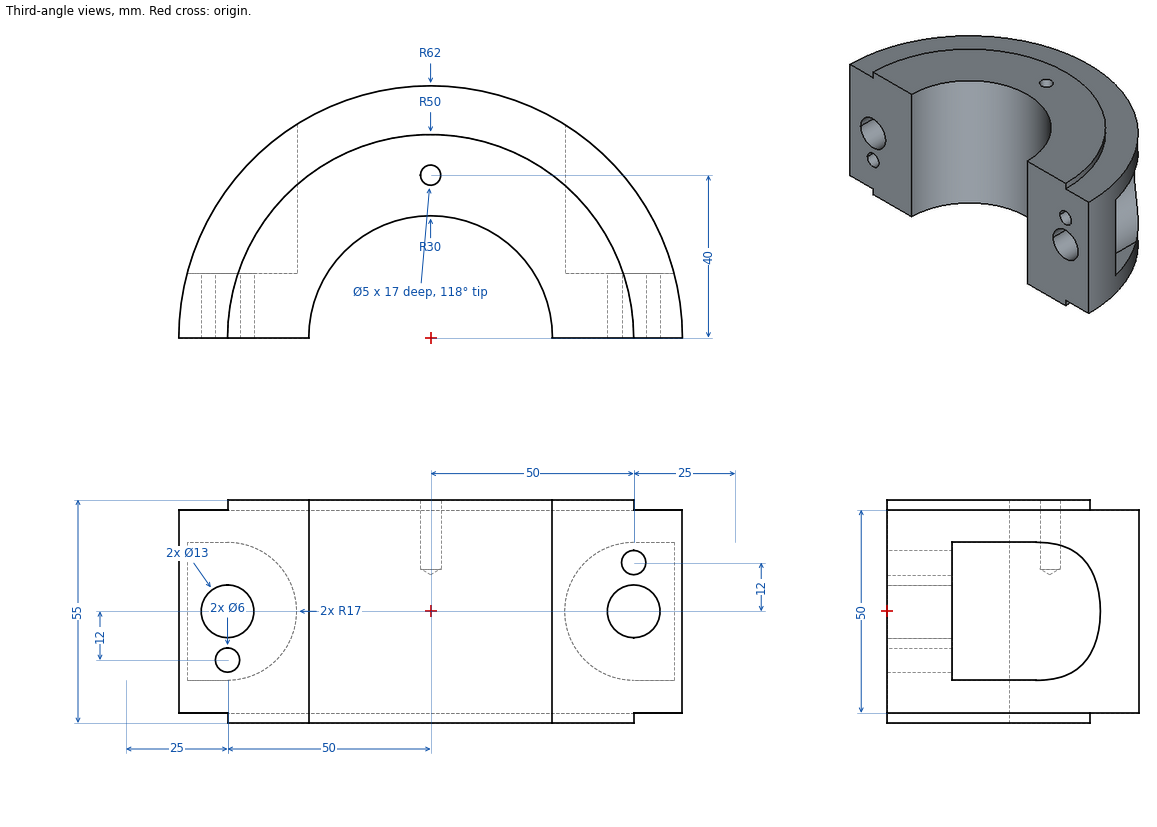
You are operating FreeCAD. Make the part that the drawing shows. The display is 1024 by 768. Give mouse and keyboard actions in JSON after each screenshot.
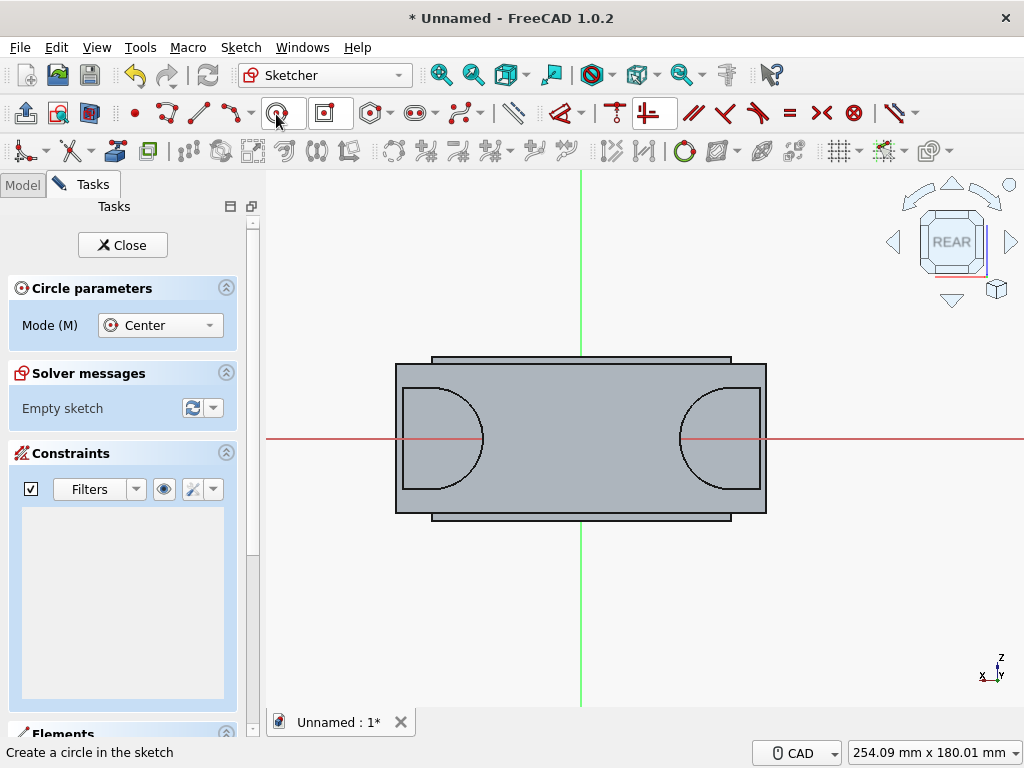
{"action": "left_click", "coordinate": [731, 439]}
{"action": "mouse_move", "coordinate": [737, 420]}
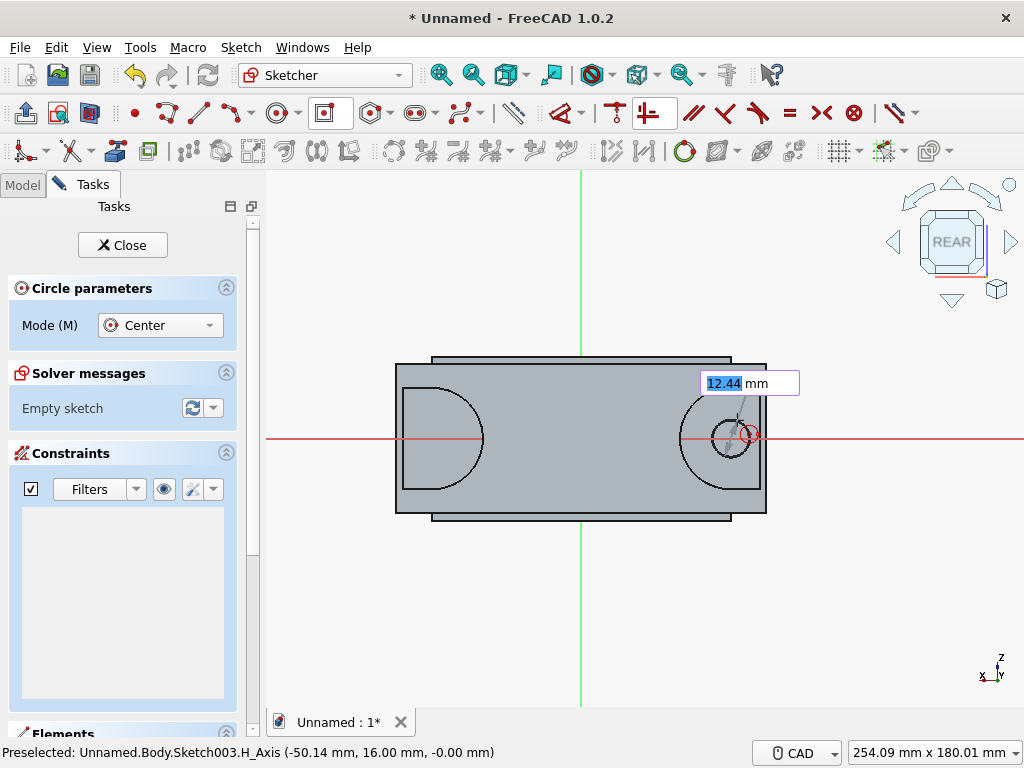
{"action": "type", "text": "13"}
{"action": "key", "text": "Return"}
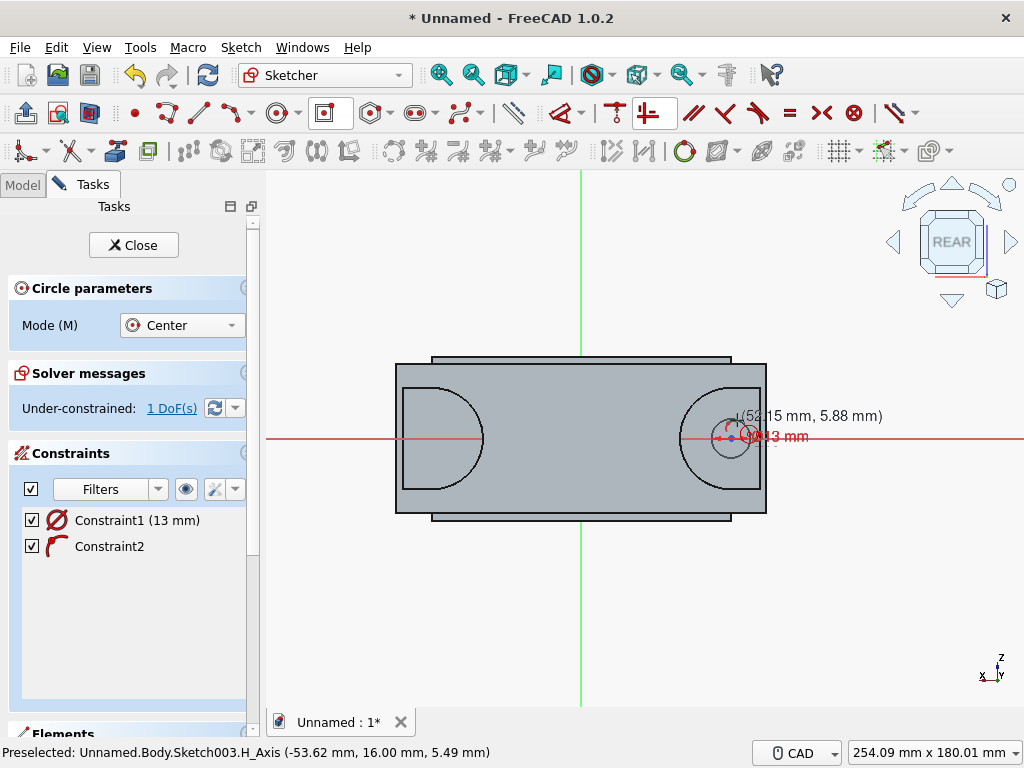
{"action": "scroll", "coordinate": [731, 474], "scroll_direction": "up", "scroll_amount": 5}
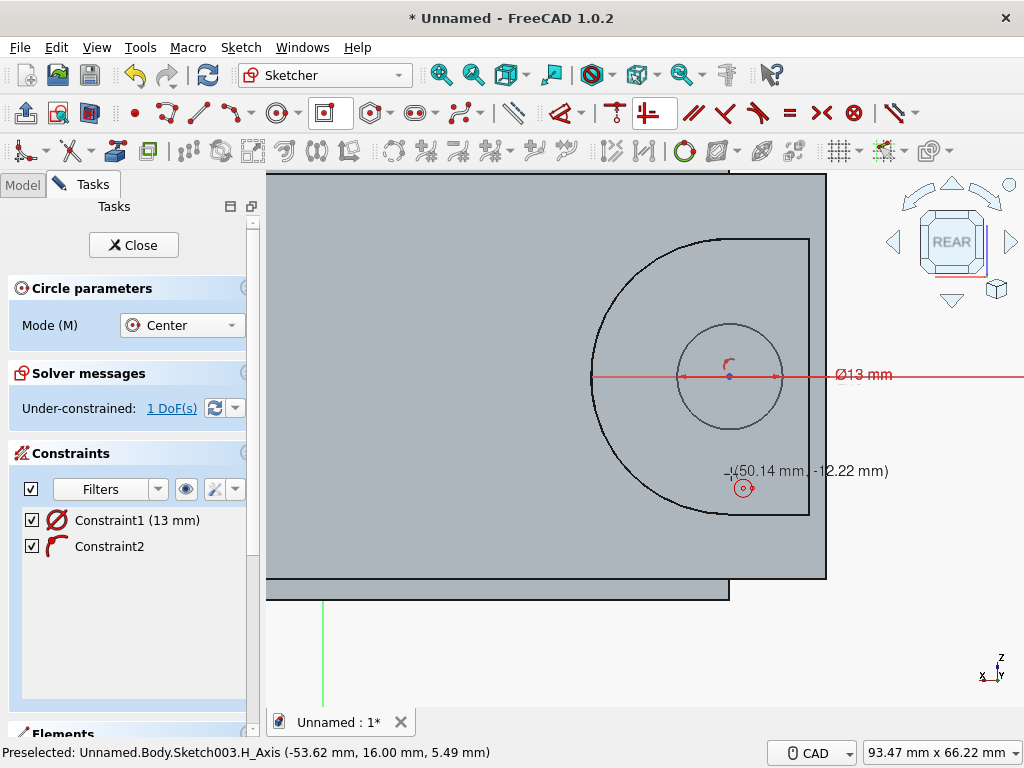
{"action": "left_click", "coordinate": [729, 474]}
{"action": "mouse_move", "coordinate": [746, 457]}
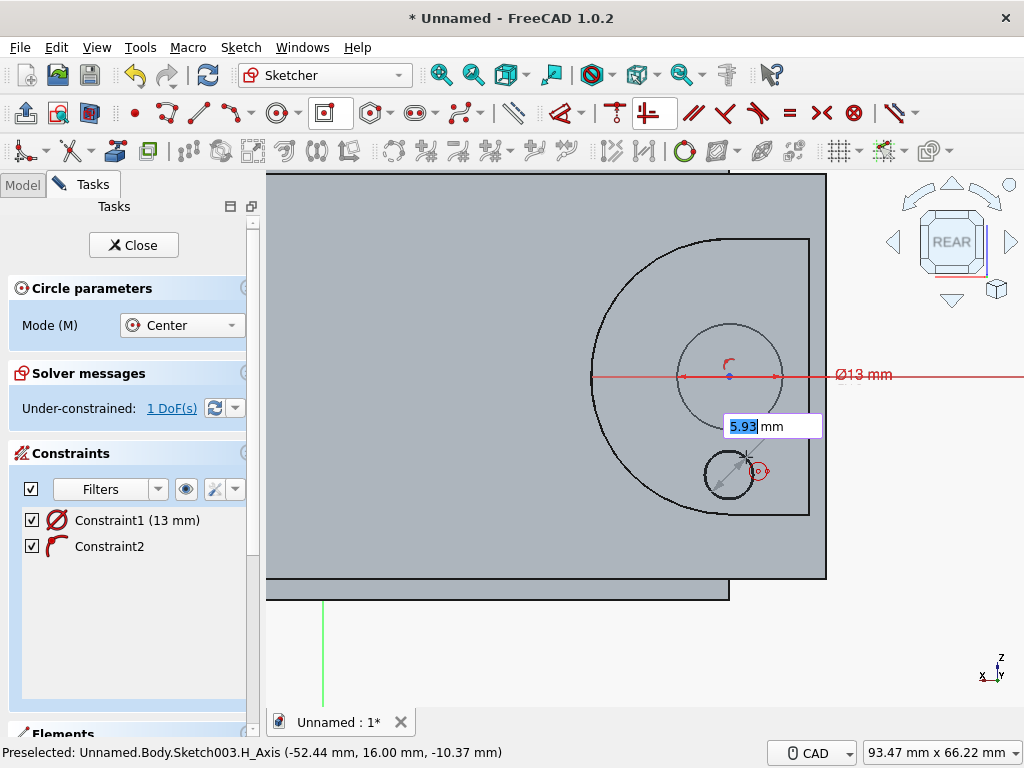
{"action": "type", "text": "6"}
{"action": "key", "text": "Return"}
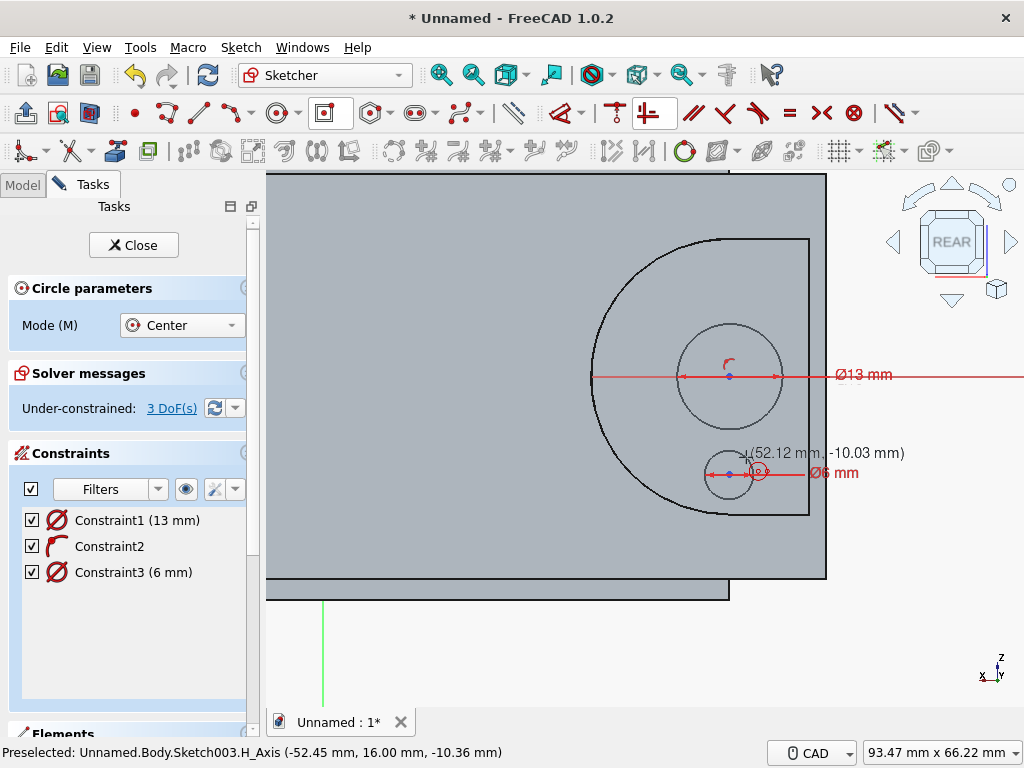
{"action": "scroll", "coordinate": [783, 489], "scroll_direction": "down", "scroll_amount": 4}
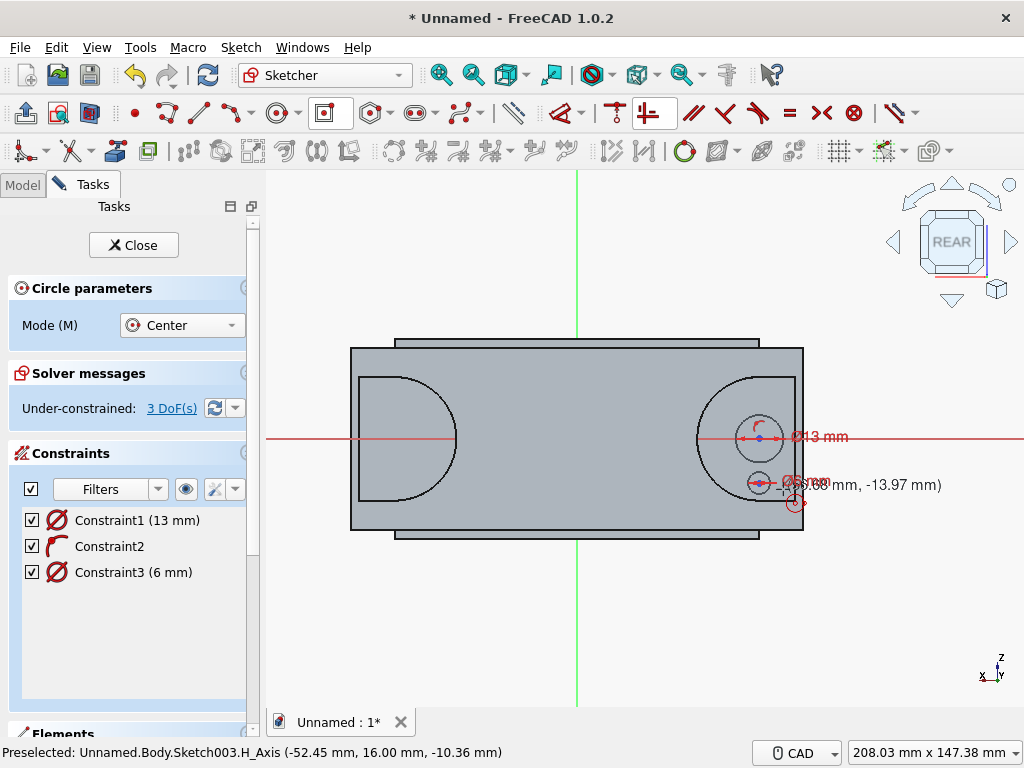
{"action": "left_click", "coordinate": [395, 439]}
{"action": "mouse_move", "coordinate": [411, 422]}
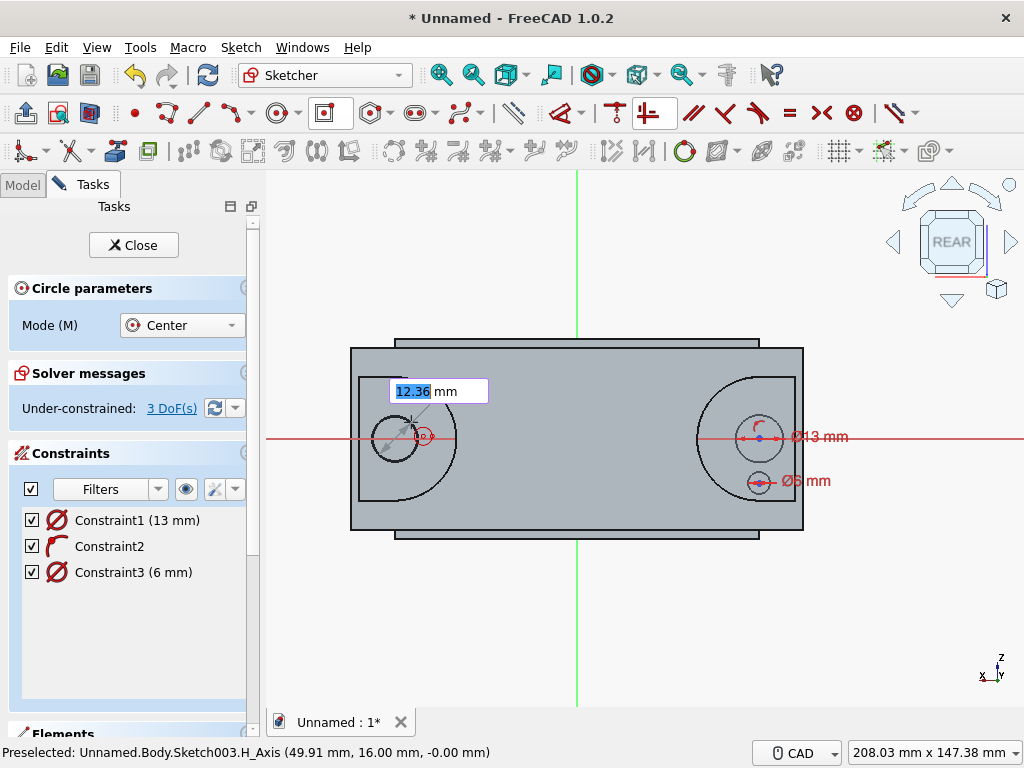
{"action": "type", "text": "13"}
{"action": "key", "text": "Return"}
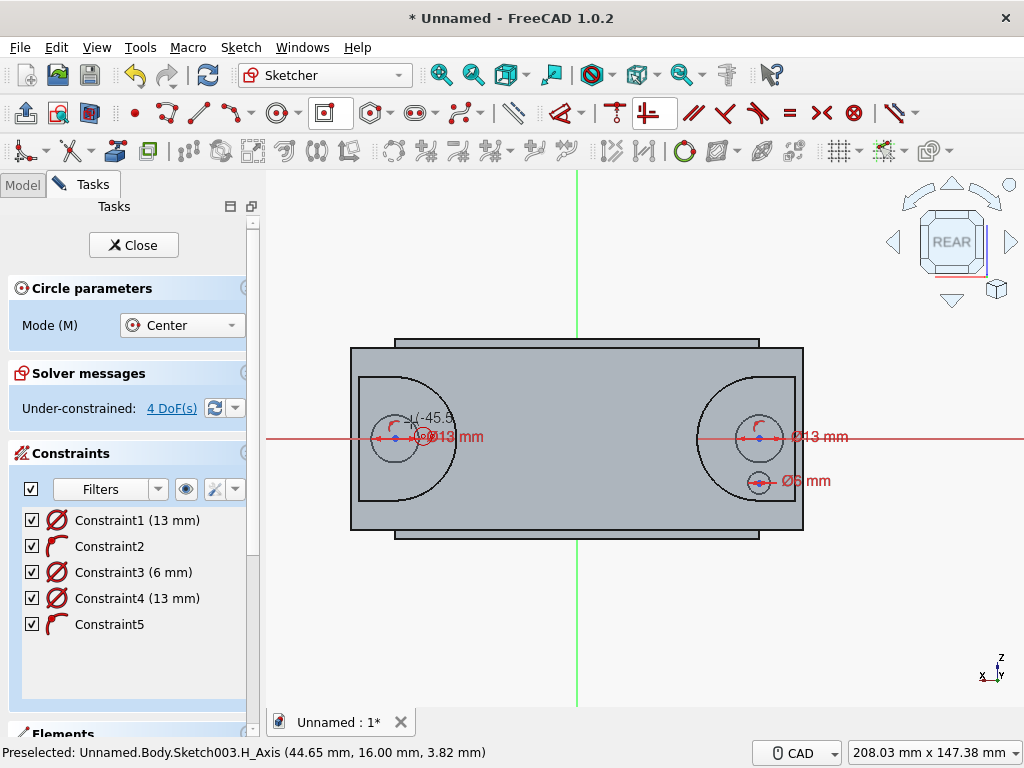
{"action": "scroll", "coordinate": [395, 395], "scroll_direction": "up", "scroll_amount": 4}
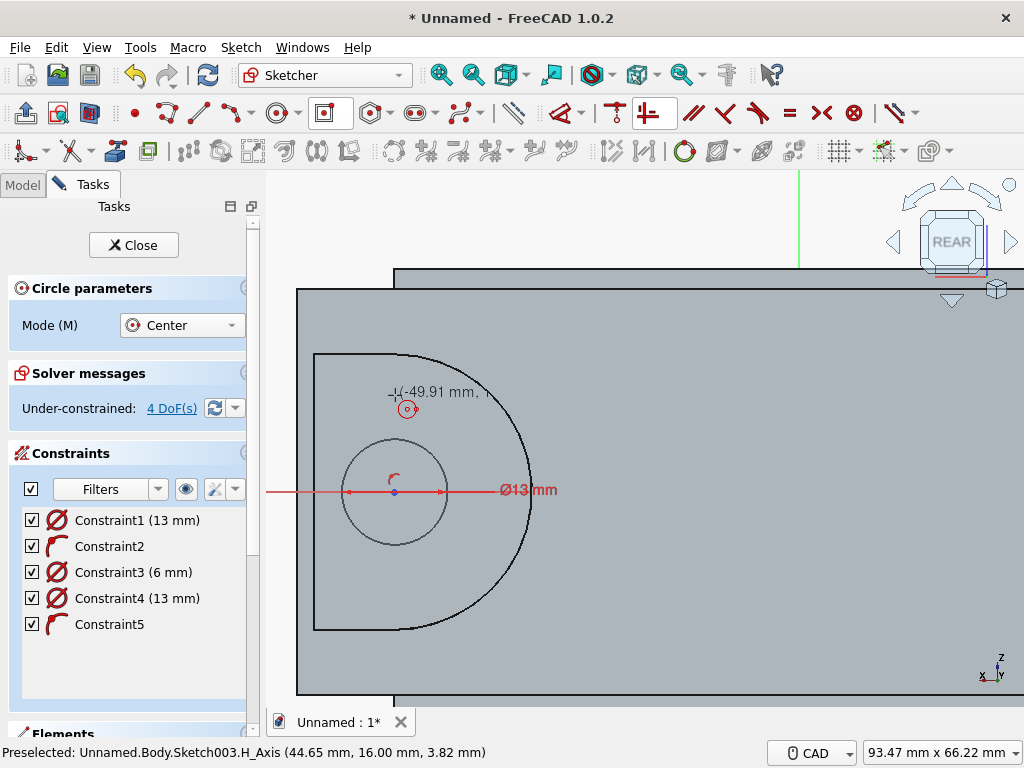
{"action": "left_click", "coordinate": [394, 395]}
{"action": "mouse_move", "coordinate": [411, 378]}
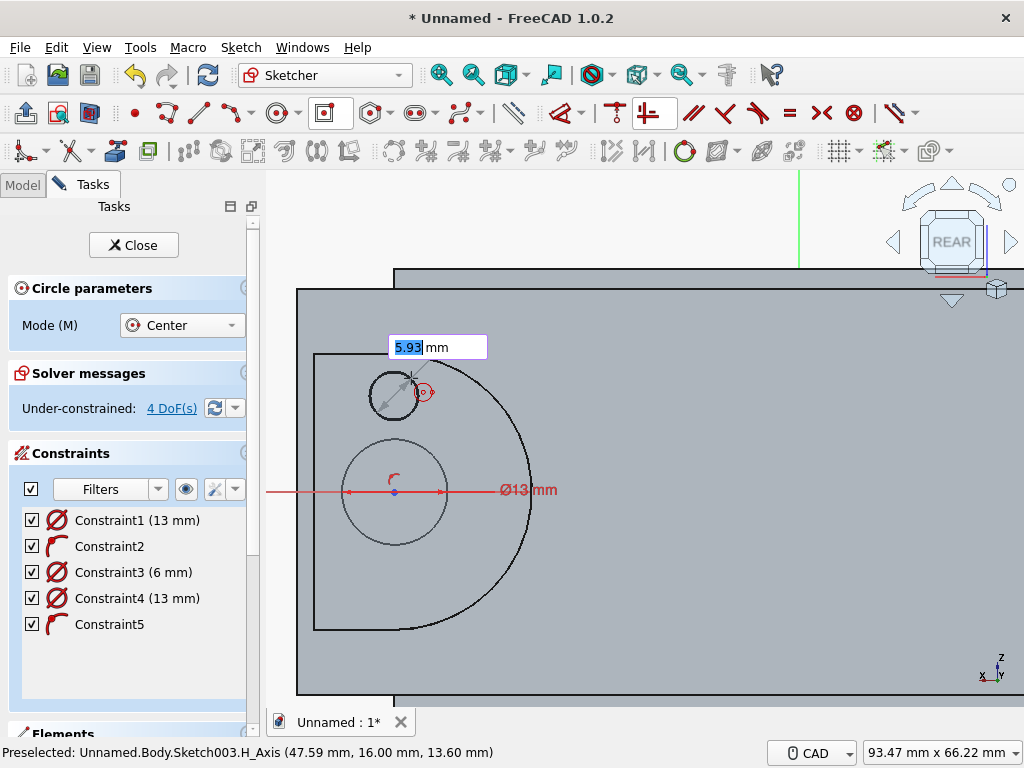
{"action": "type", "text": "6"}
{"action": "key", "text": "Return"}
{"action": "key", "text": "Escape"}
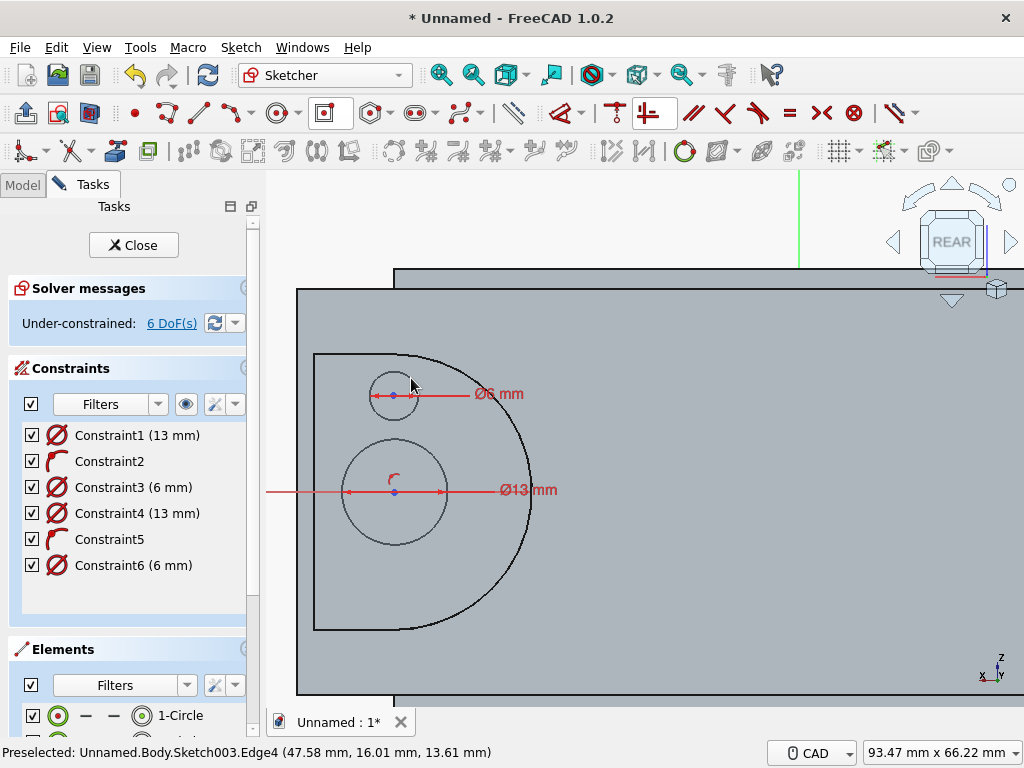
{"action": "scroll", "coordinate": [395, 395], "scroll_direction": "down", "scroll_amount": 4}